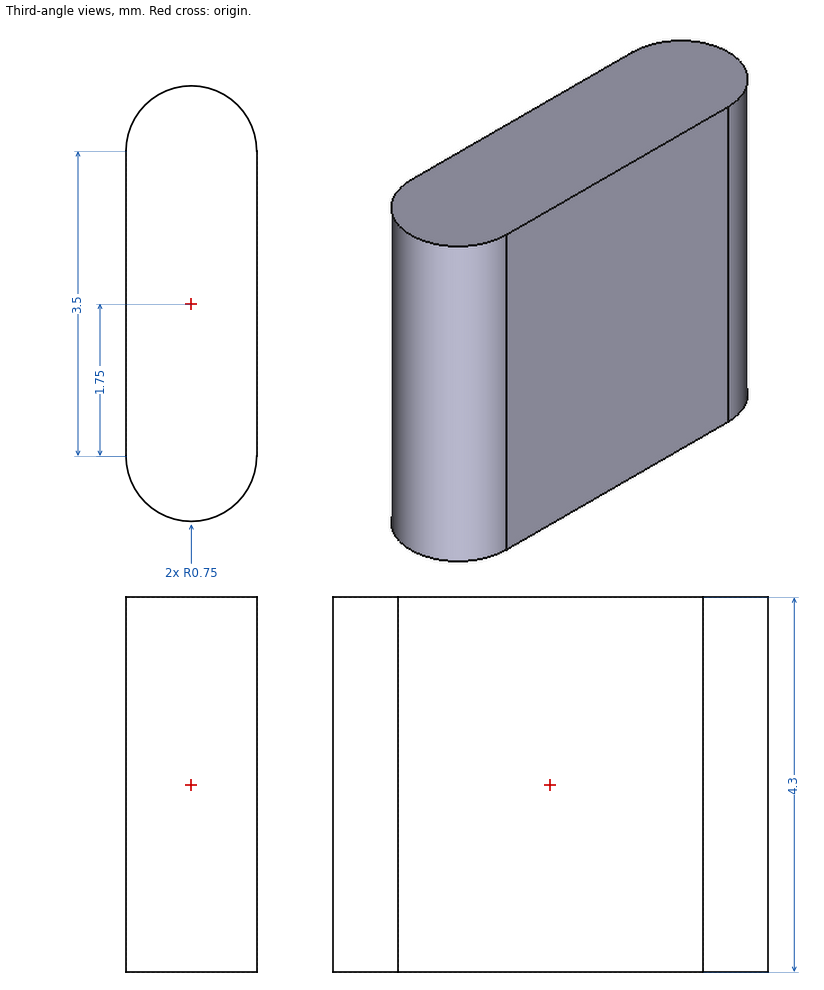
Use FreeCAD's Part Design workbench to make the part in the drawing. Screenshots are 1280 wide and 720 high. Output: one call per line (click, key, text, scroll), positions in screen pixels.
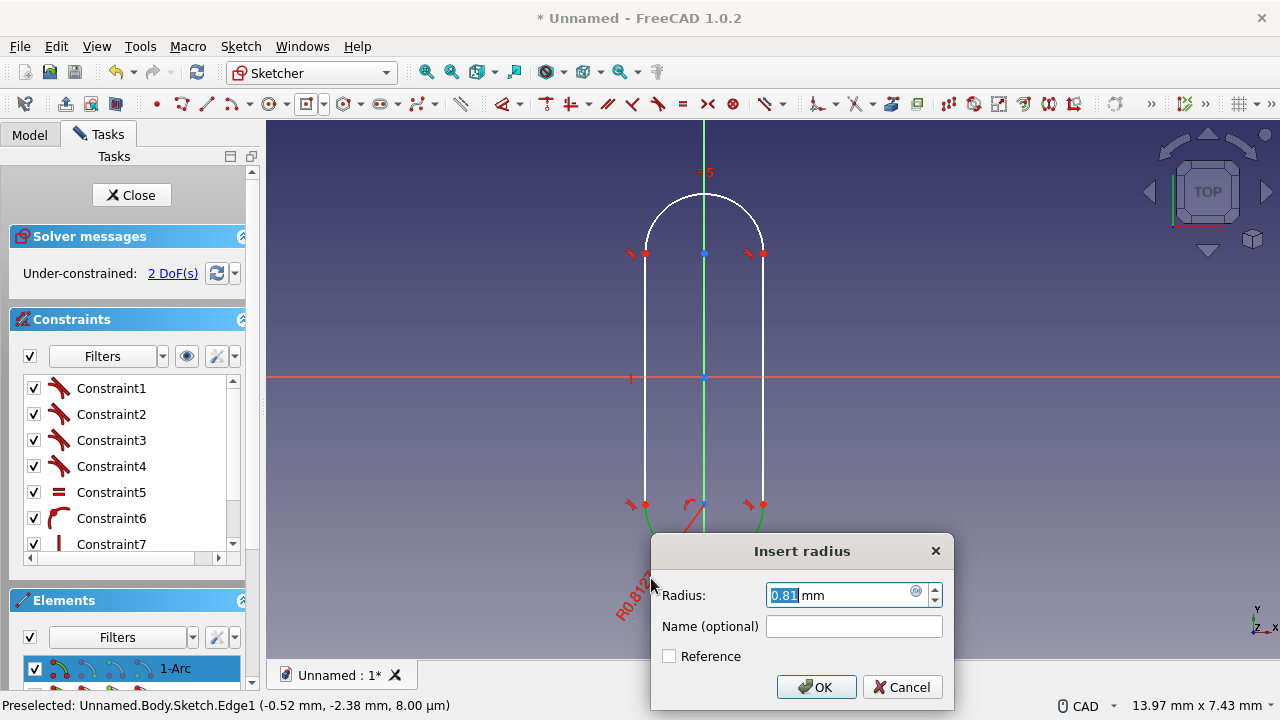
text(0.75)
key(Return)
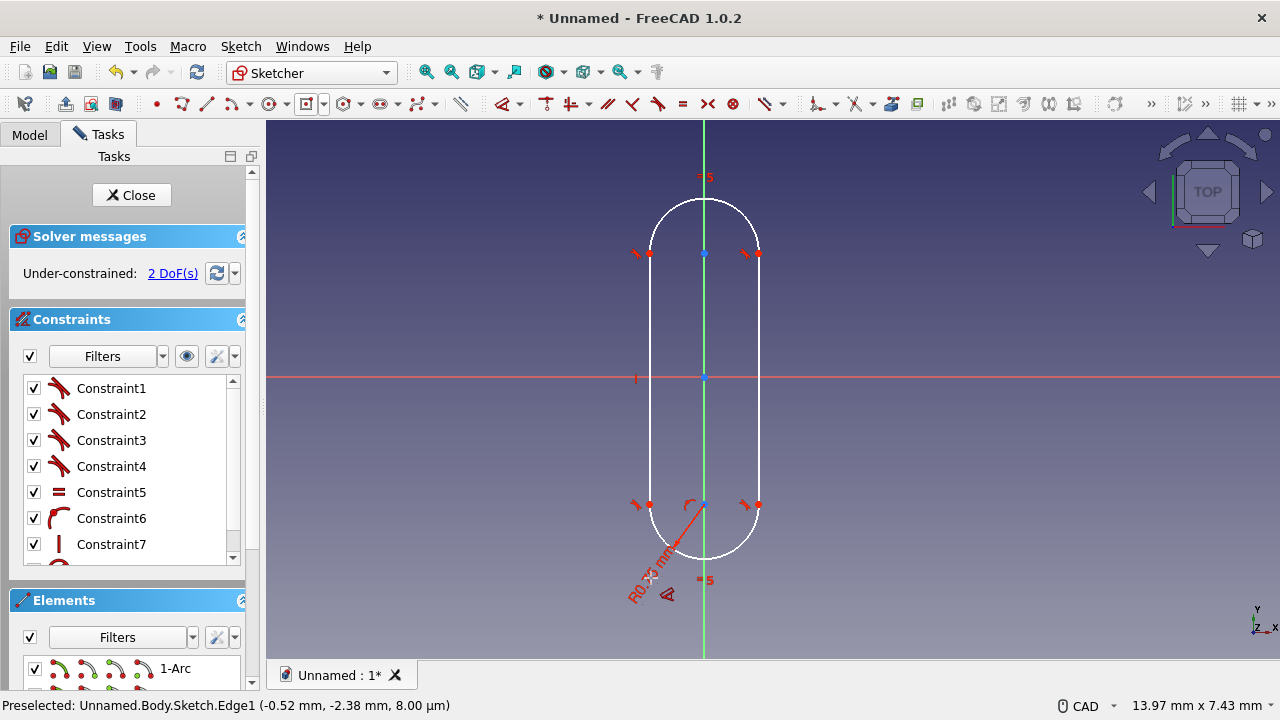
click(650, 429)
click(616, 321)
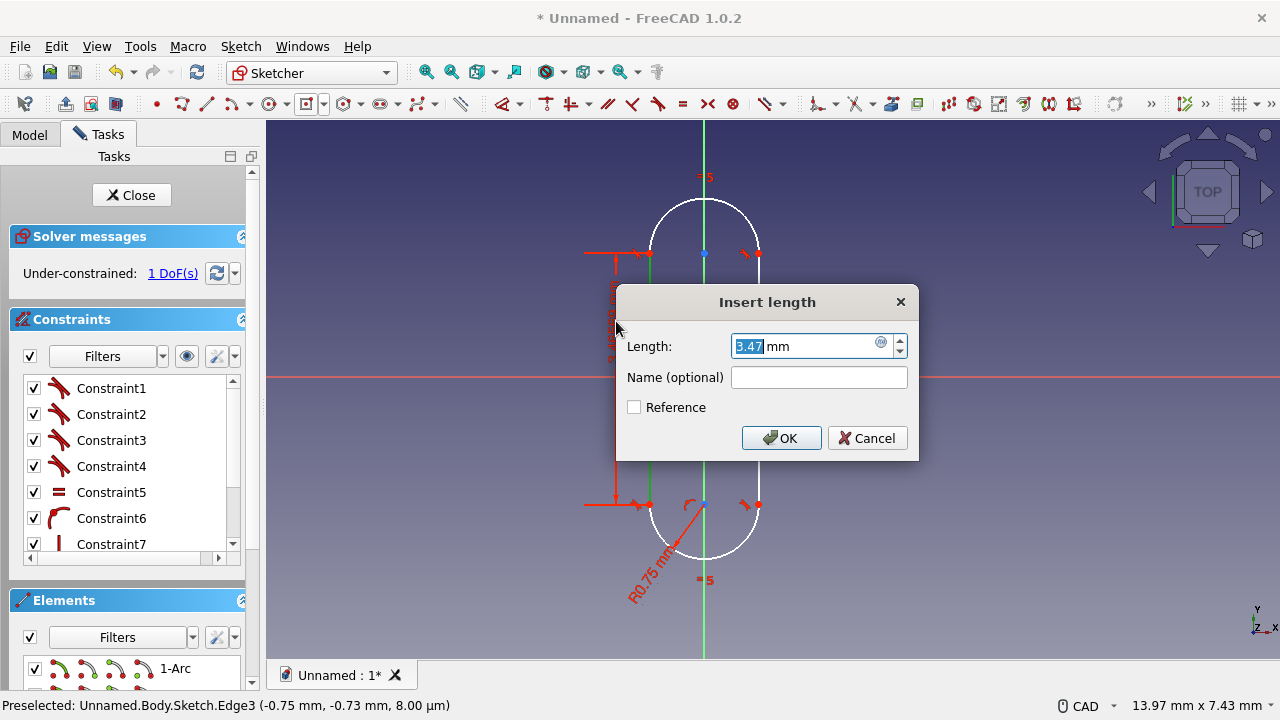
text(3.5)
key(Return)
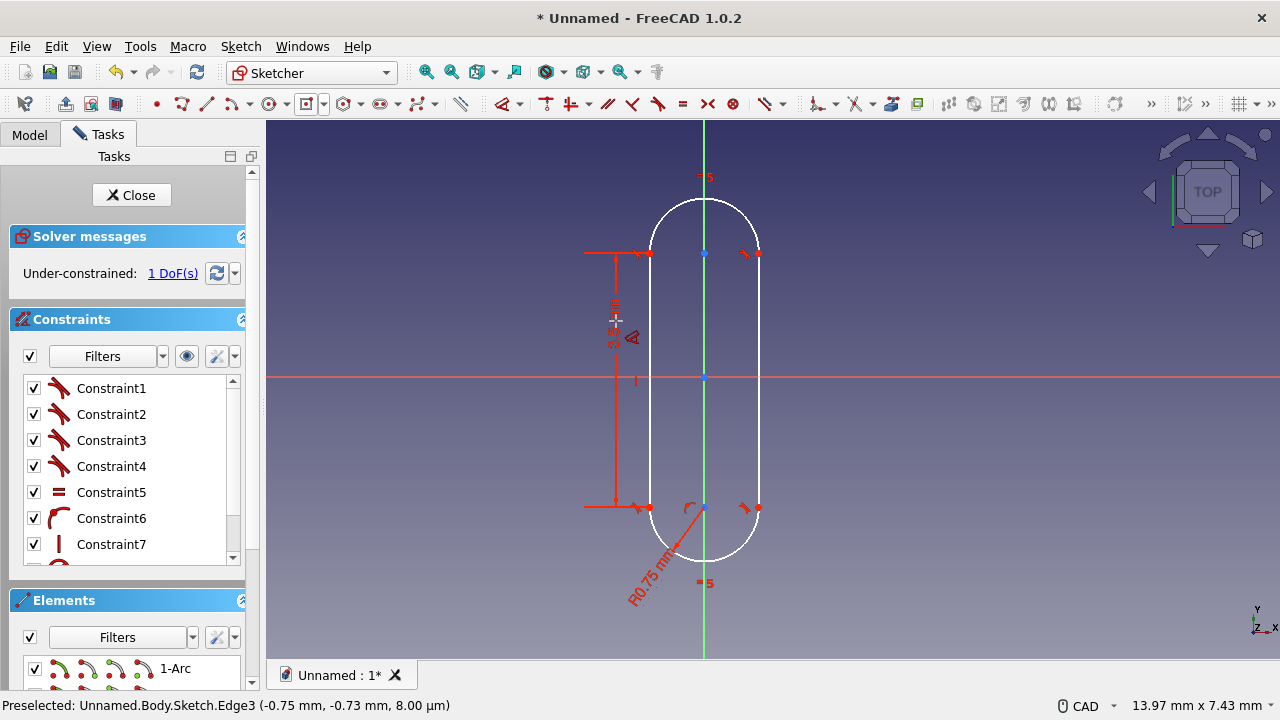
click(650, 507)
click(616, 442)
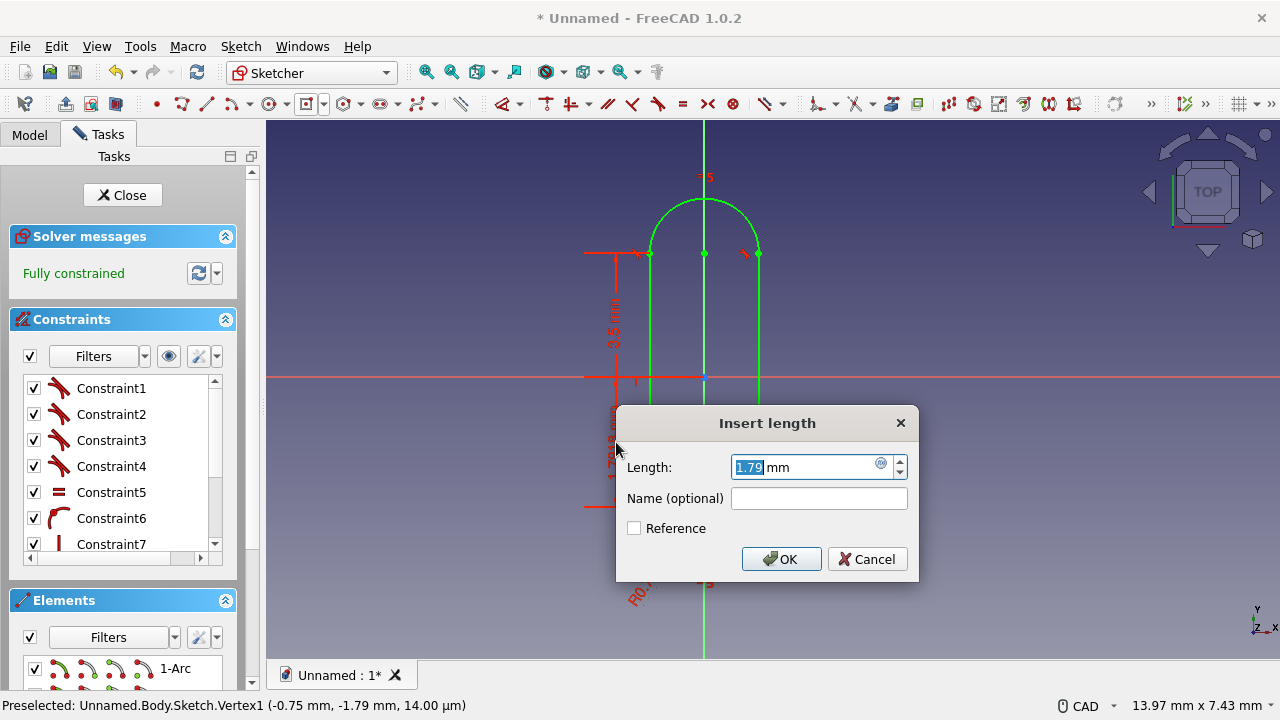
text(1.75)
key(Return)
key(Escape)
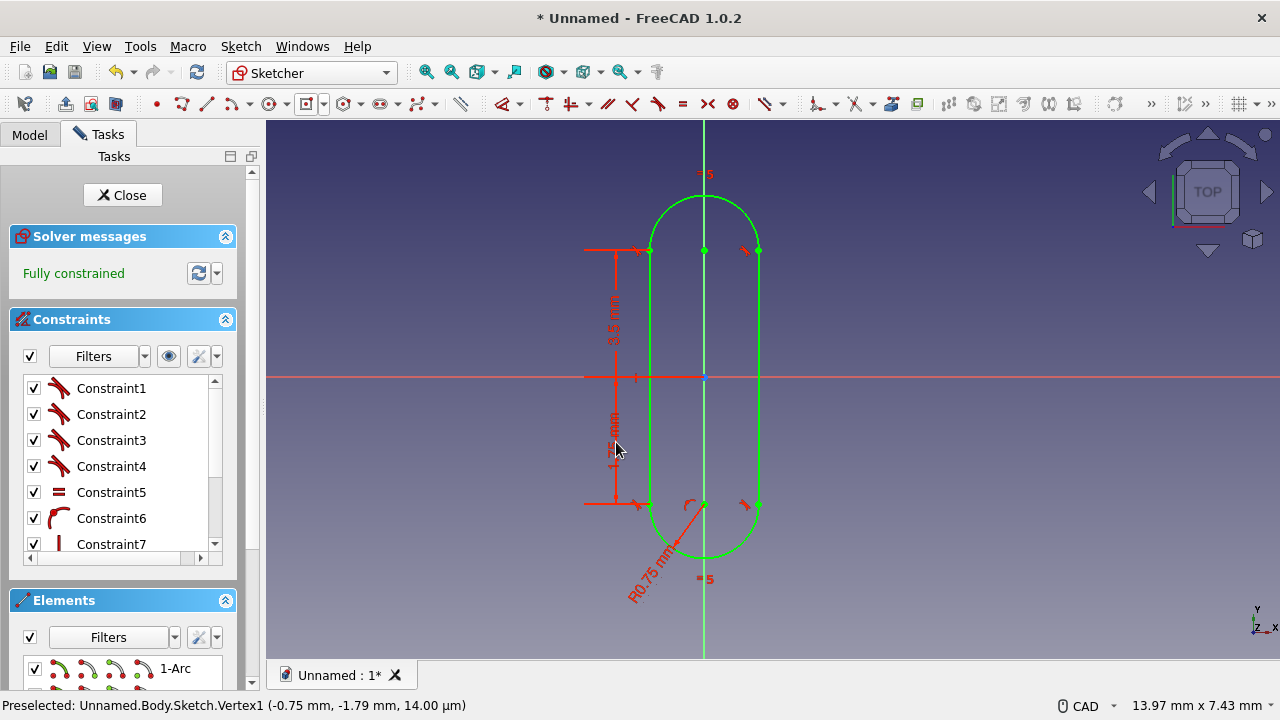
click(123, 195)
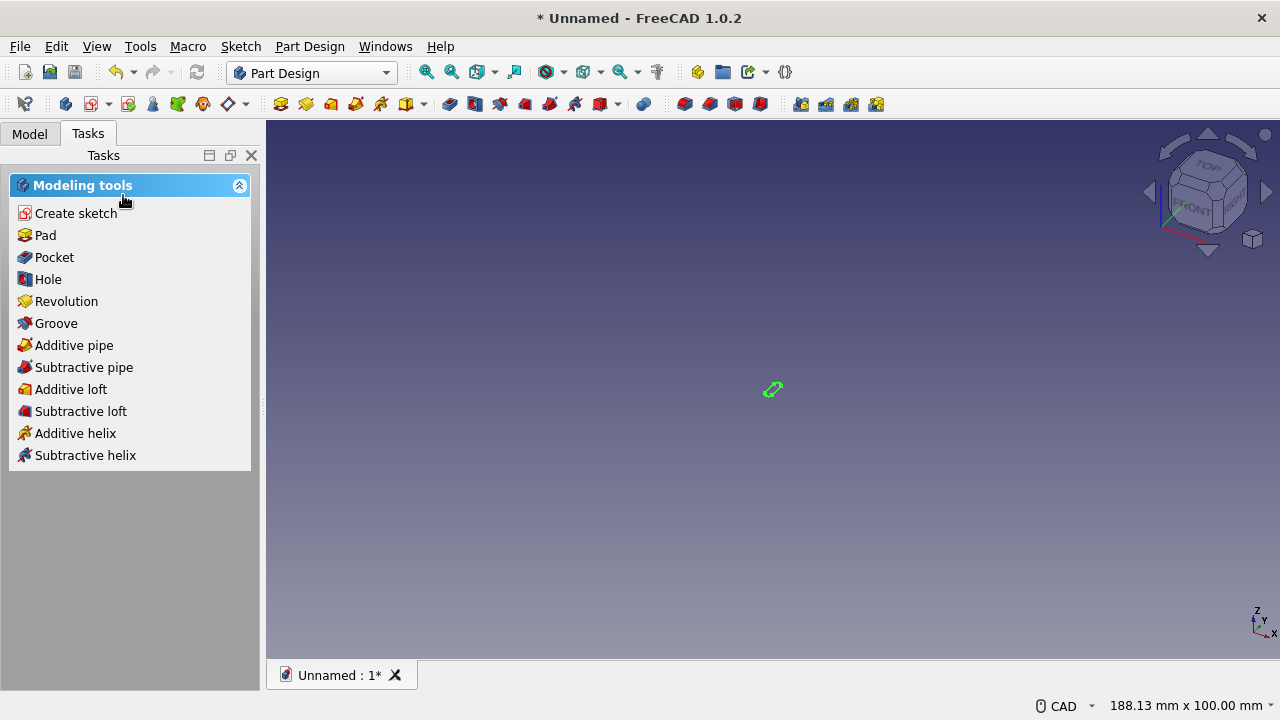
click(281, 104)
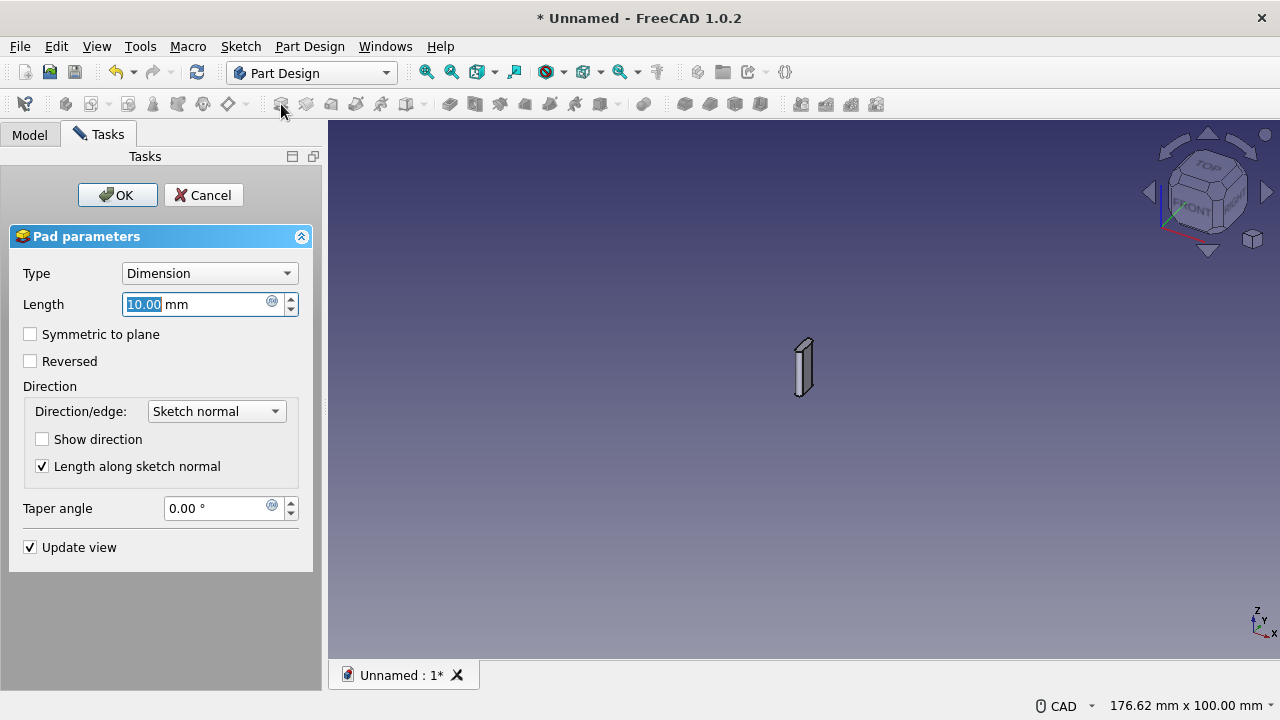
text(4.3)
key(Tab)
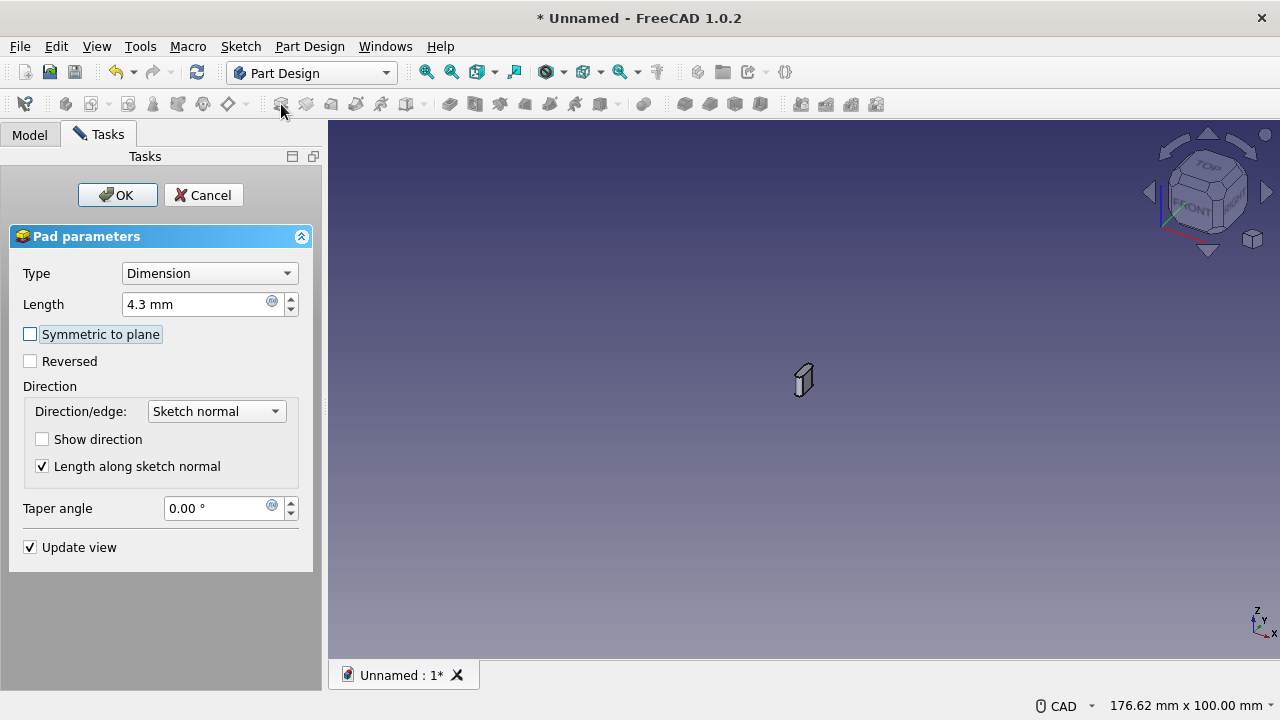
click(31, 334)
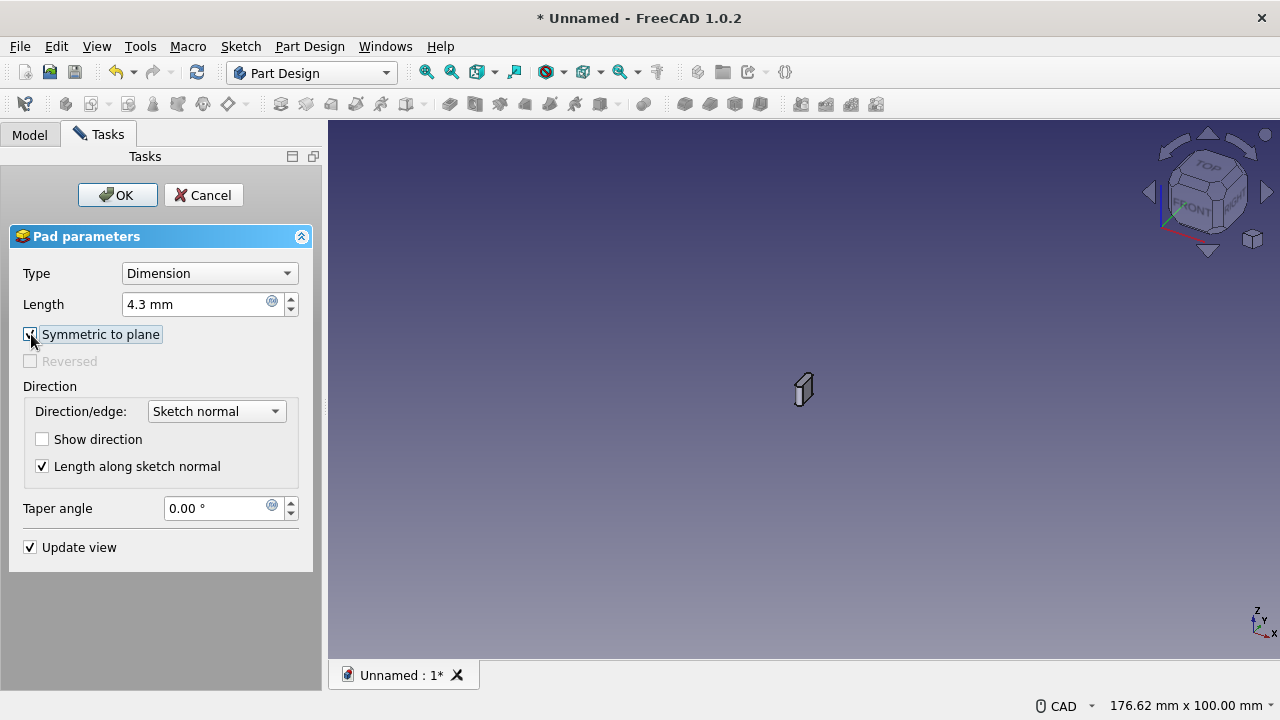
click(118, 195)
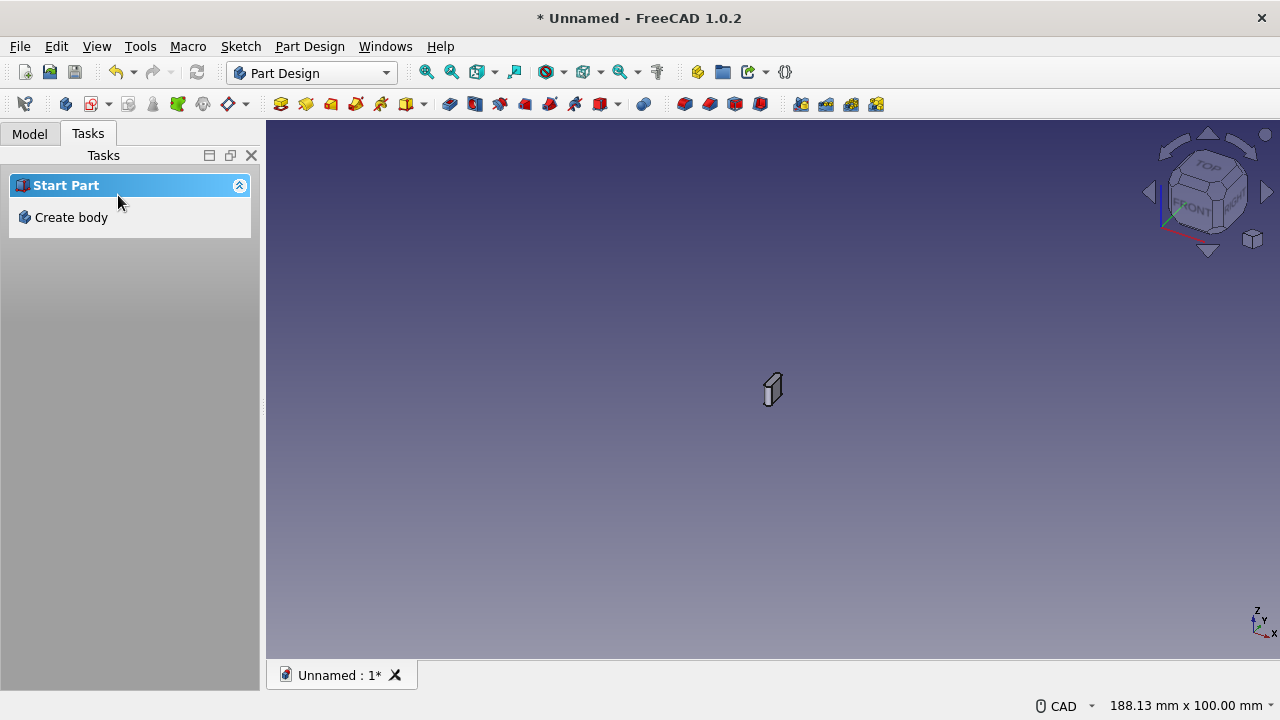
key(0)